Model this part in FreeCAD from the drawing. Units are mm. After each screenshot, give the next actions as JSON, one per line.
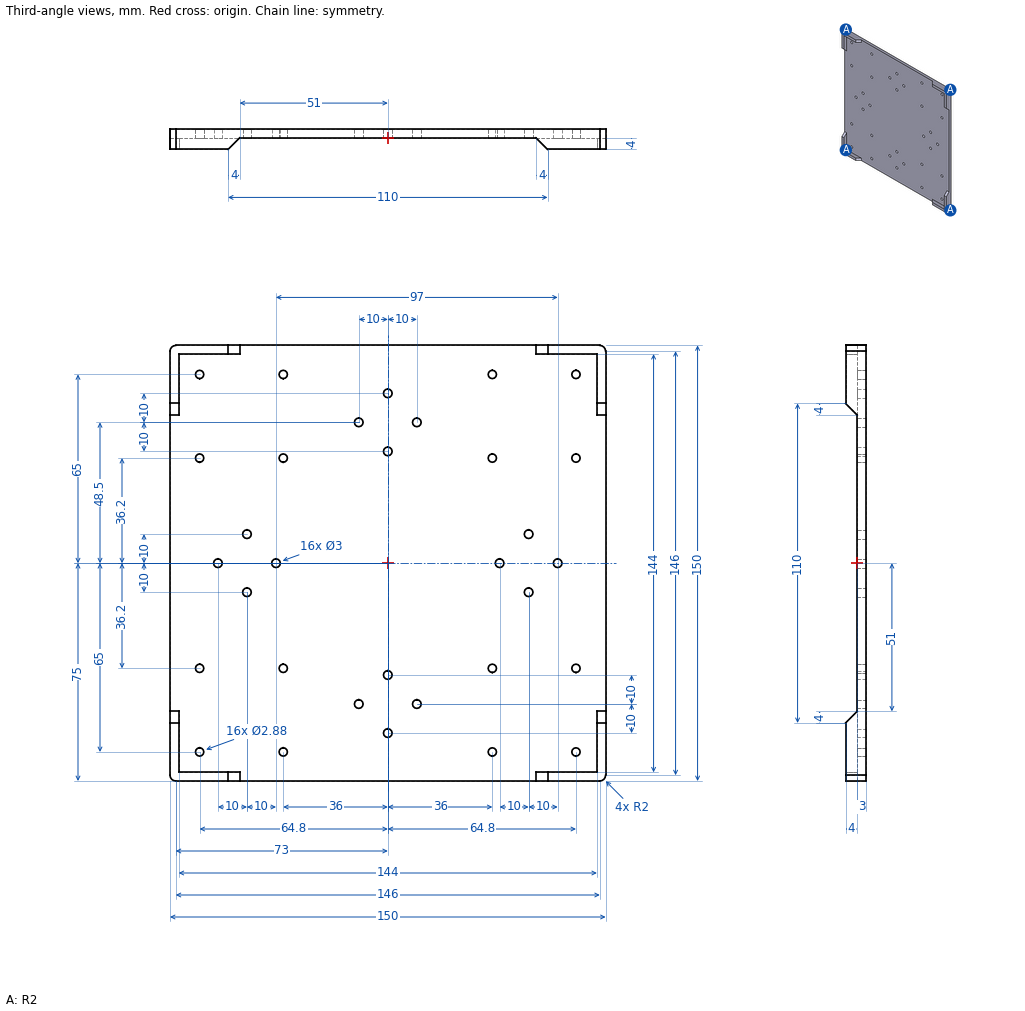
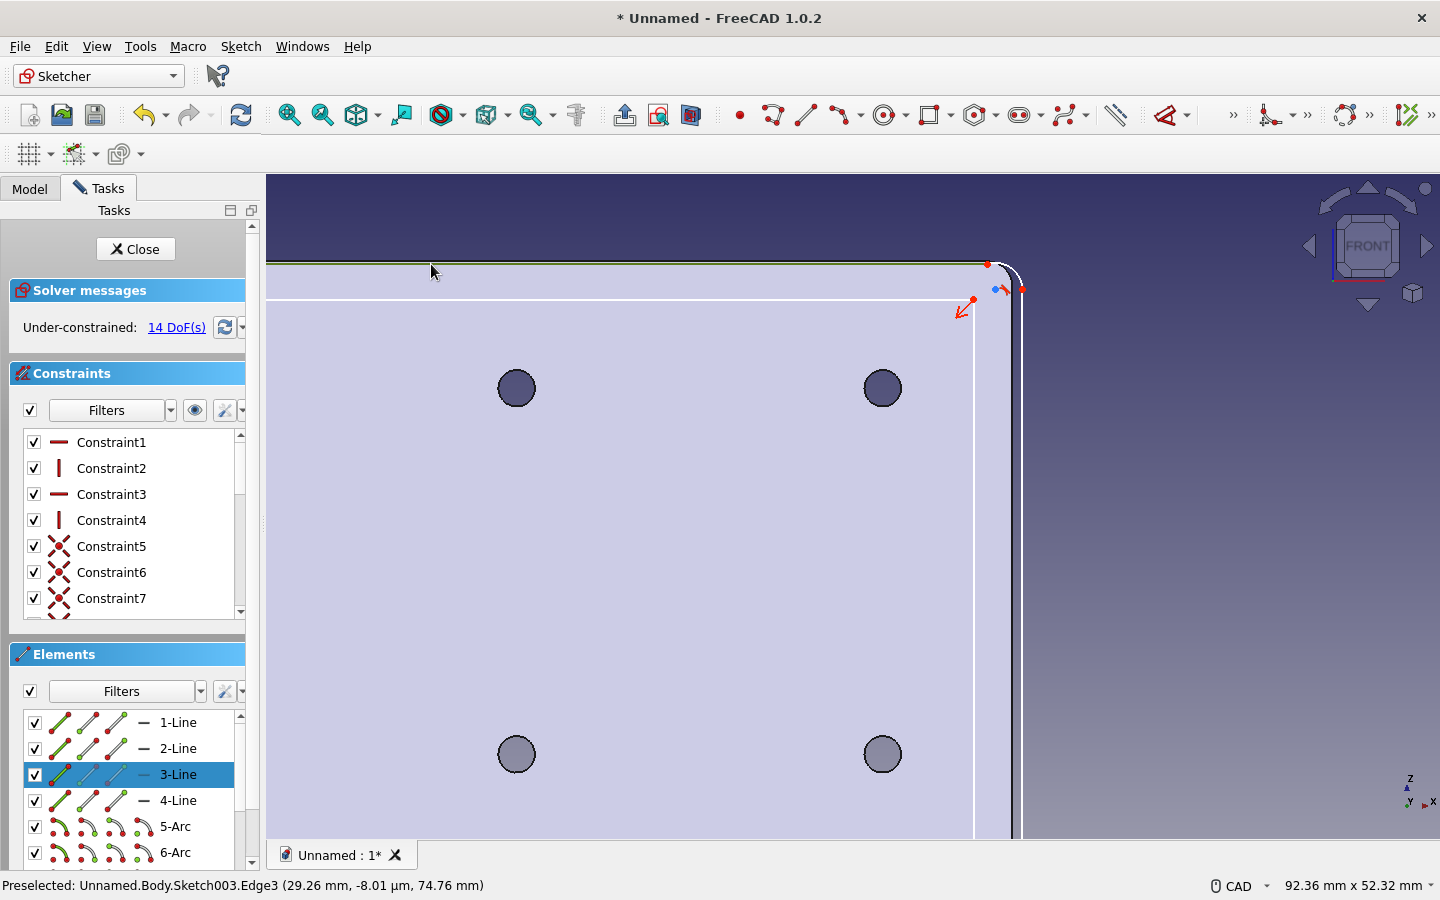
{"action": "left_click", "coordinate": [1018, 276]}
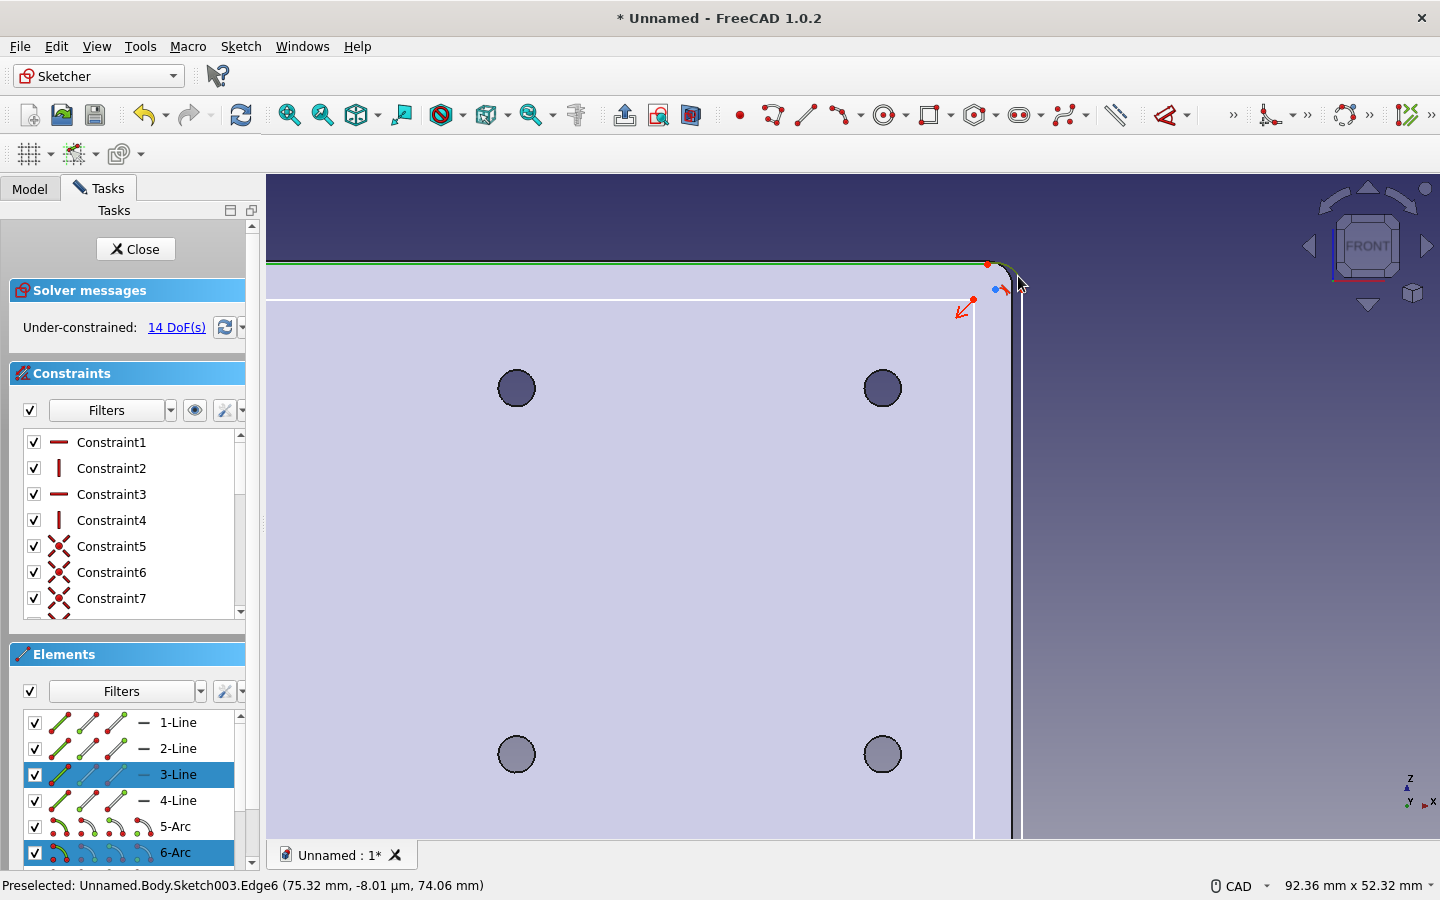
{"action": "key", "text": "t"}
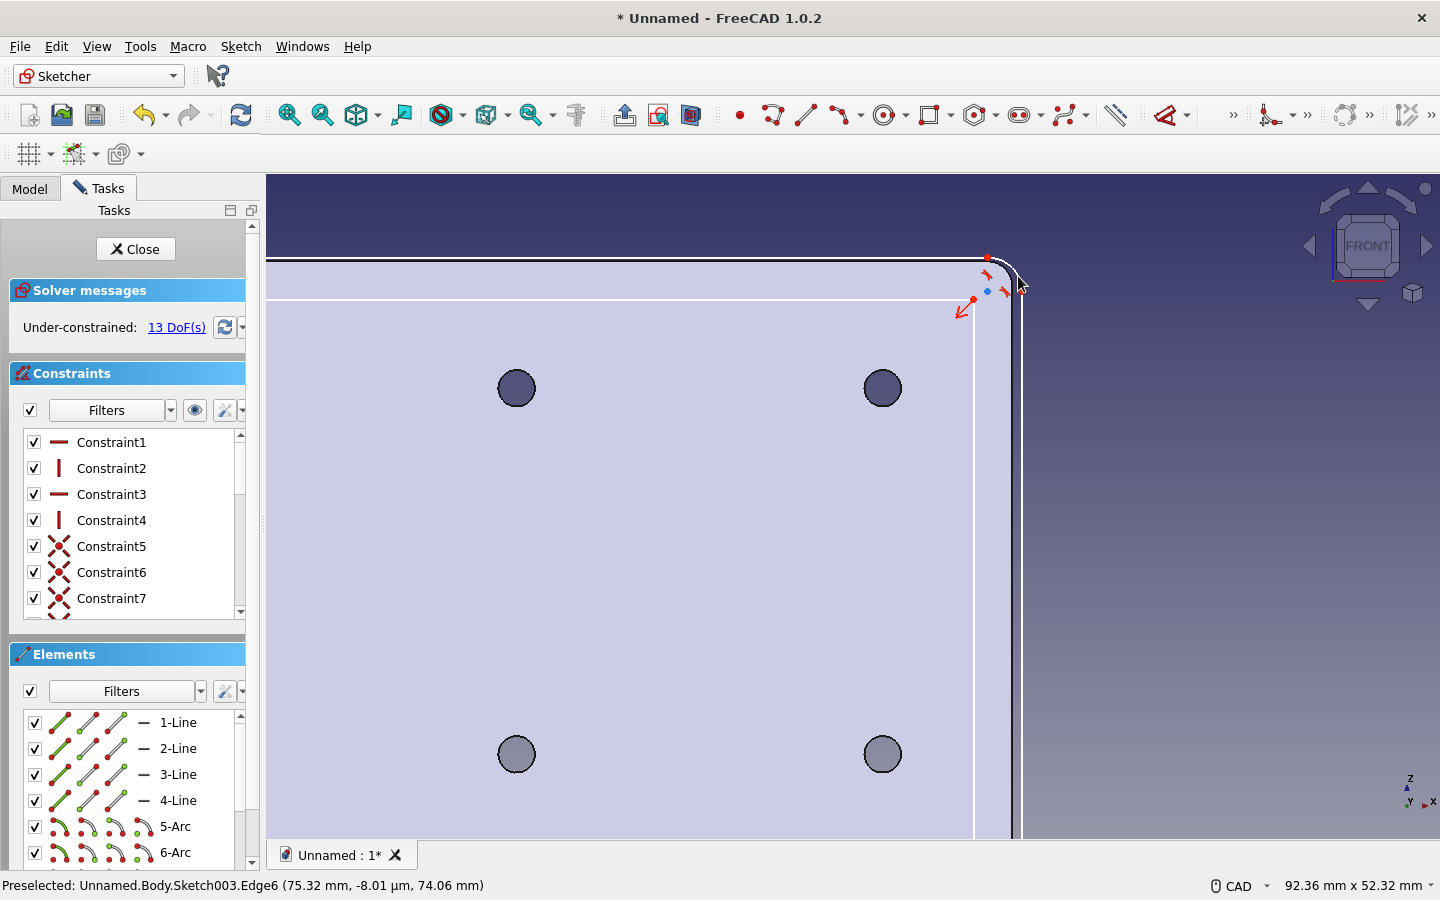
{"action": "scroll", "coordinate": [1022, 275], "scroll_direction": "down", "scroll_amount": 7}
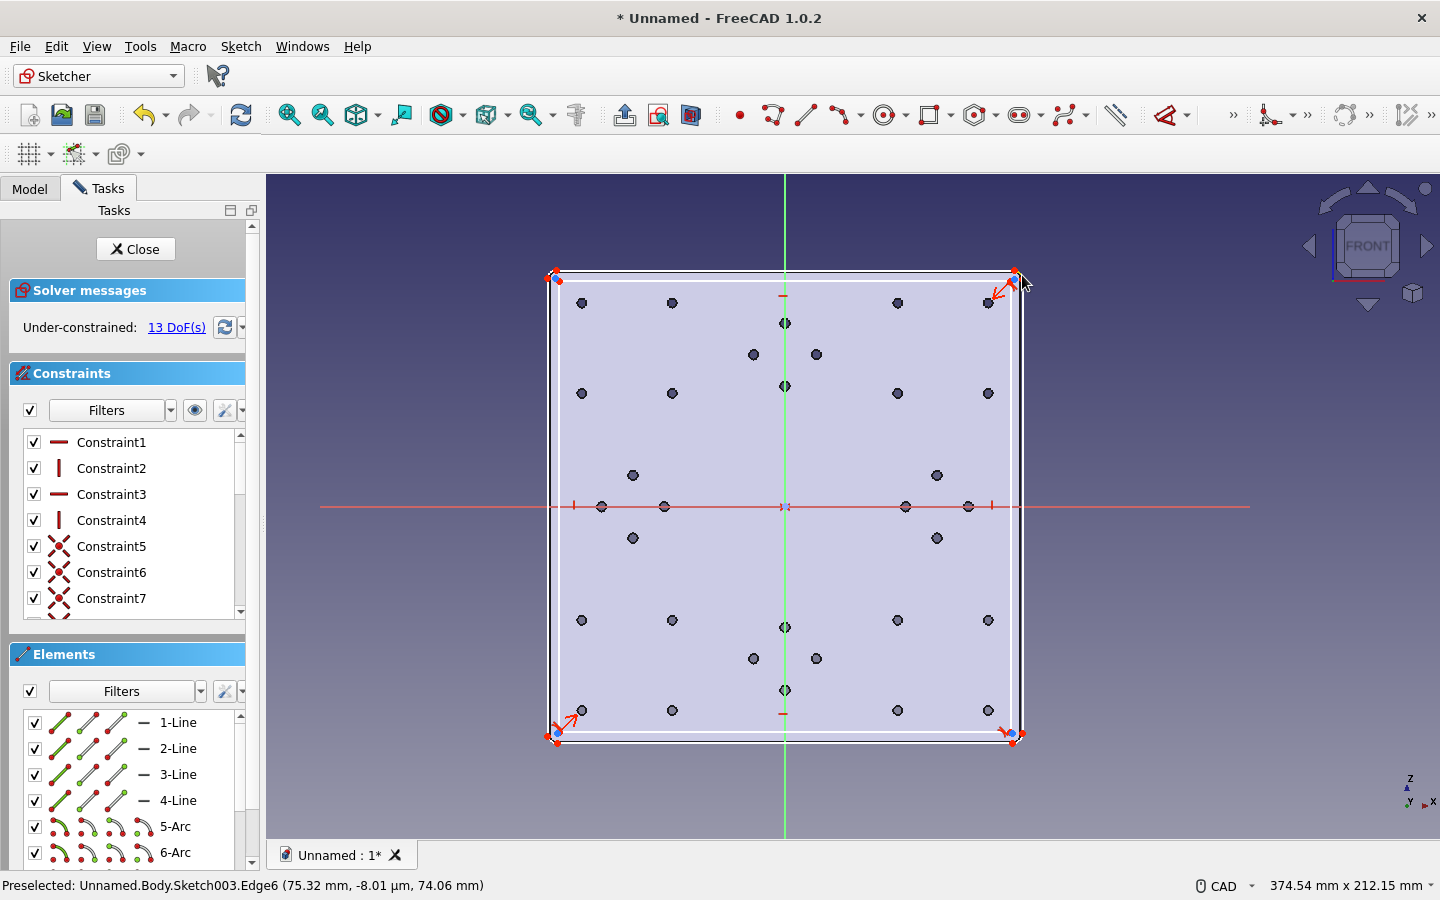
{"action": "scroll", "coordinate": [877, 271], "scroll_direction": "up", "scroll_amount": 2}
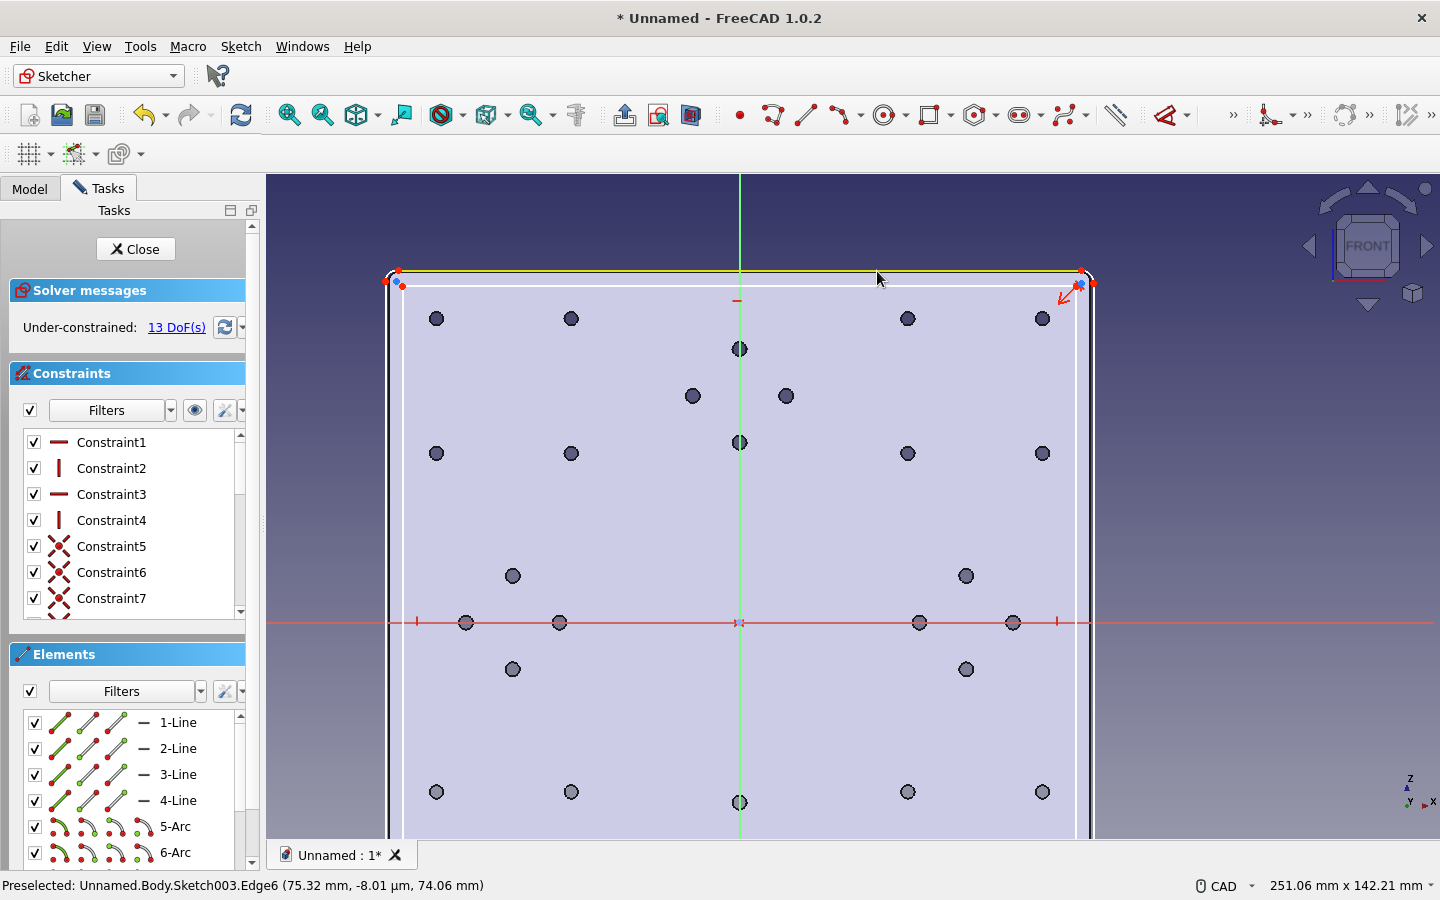
{"action": "left_click", "coordinate": [876, 271]}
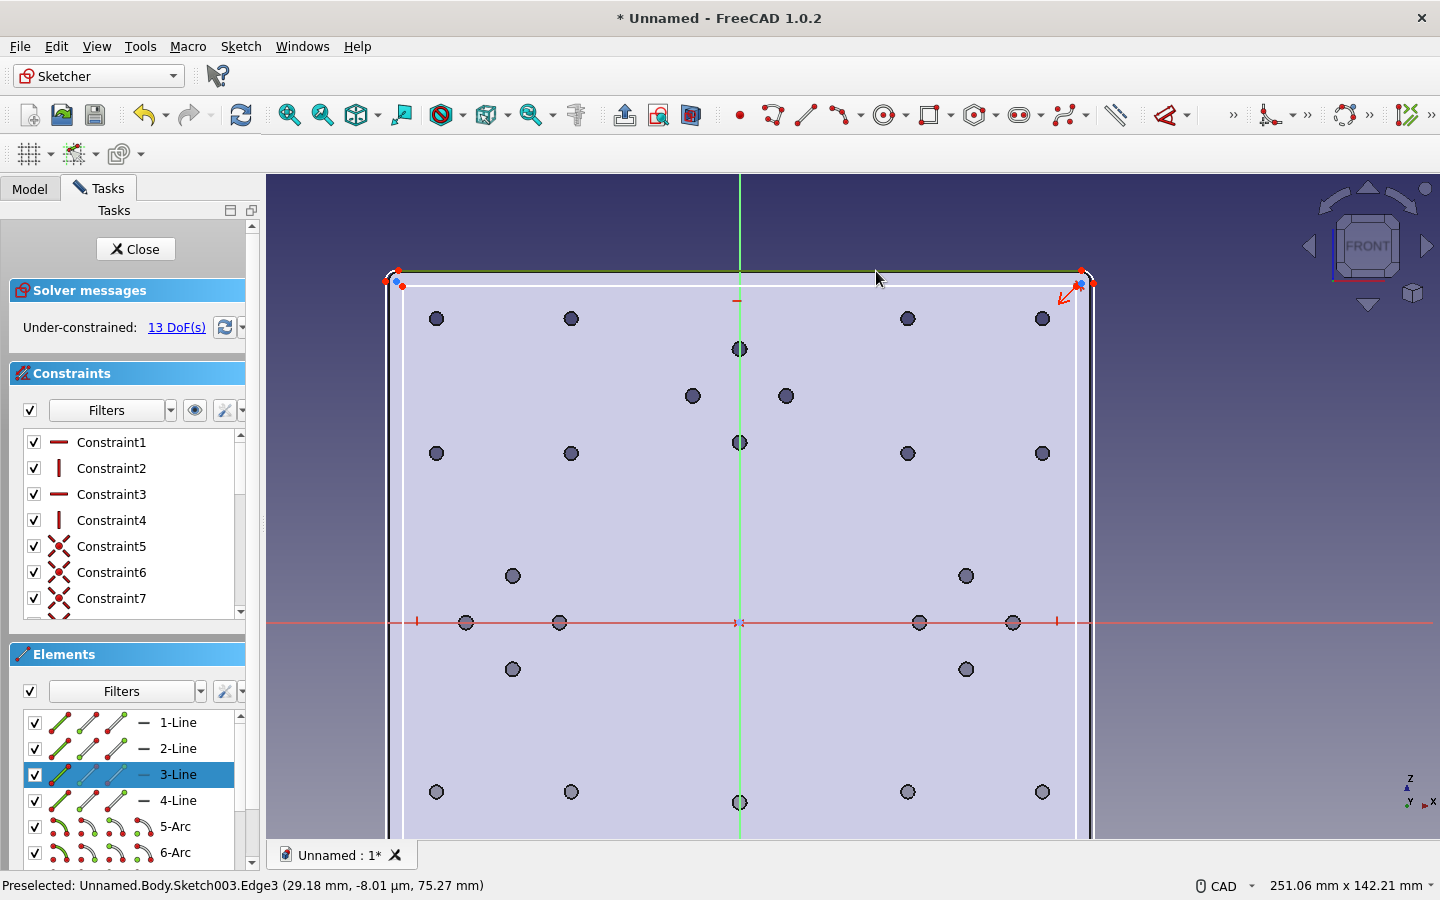
{"action": "scroll", "coordinate": [389, 273], "scroll_direction": "up", "scroll_amount": 2}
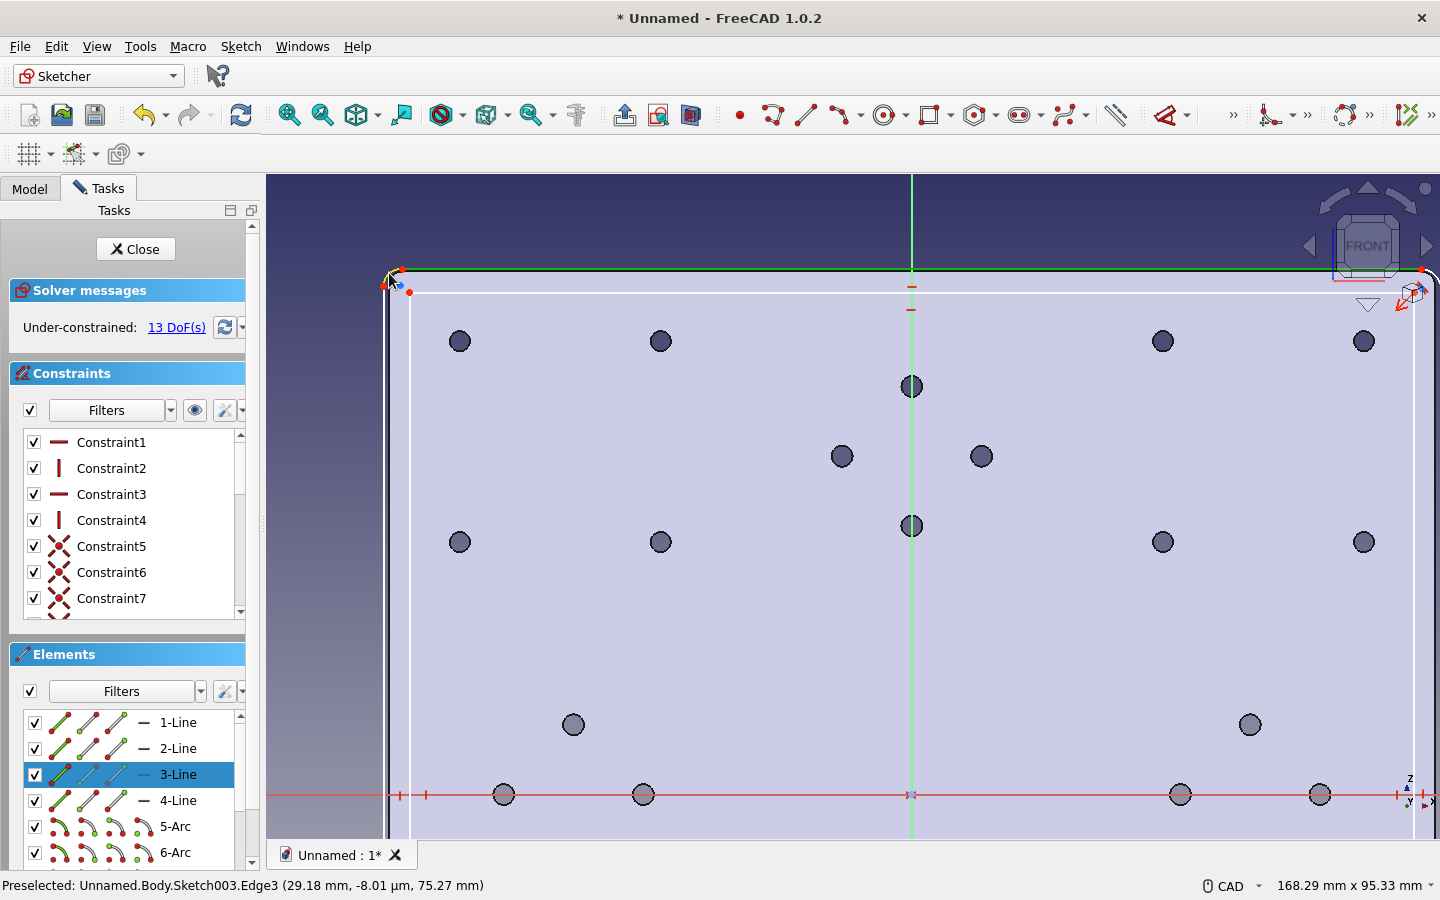
{"action": "left_click", "coordinate": [389, 273]}